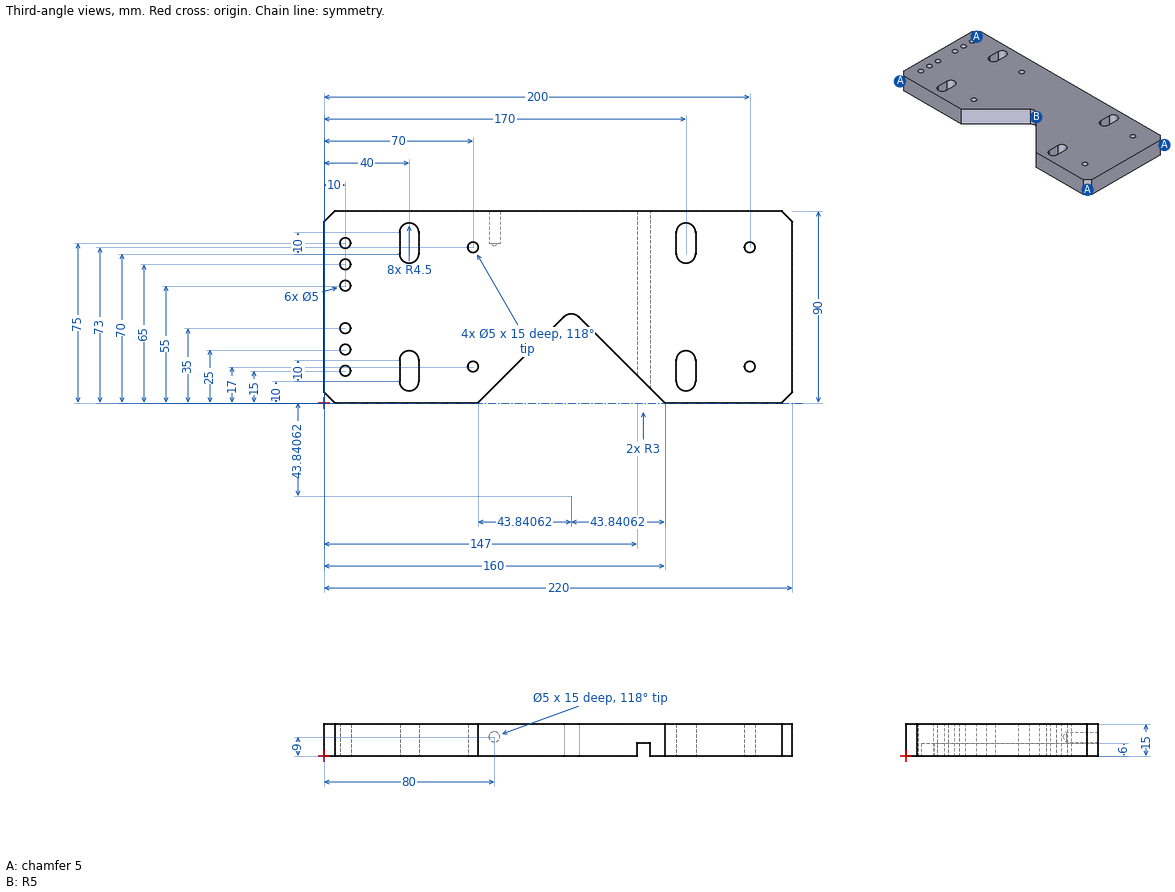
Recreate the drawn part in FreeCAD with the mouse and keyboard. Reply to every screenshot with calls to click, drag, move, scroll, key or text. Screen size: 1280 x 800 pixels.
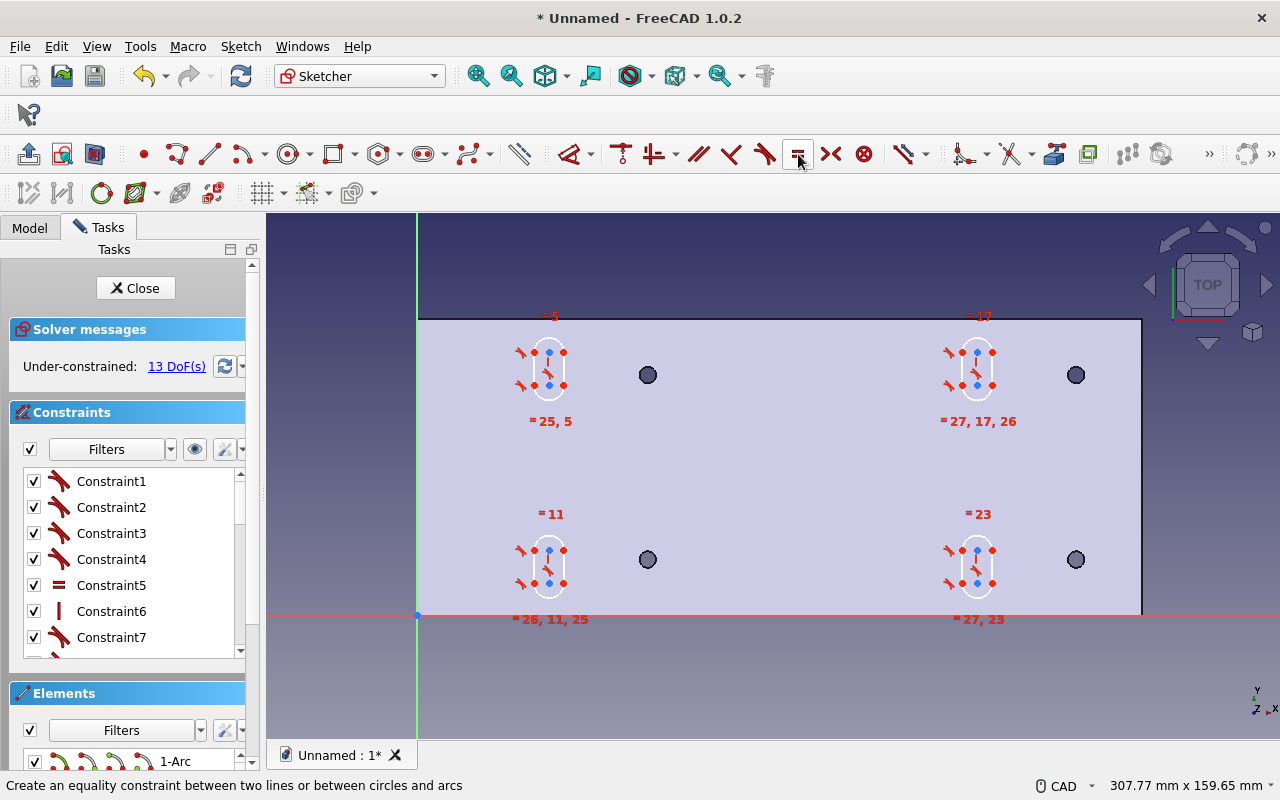
key(d)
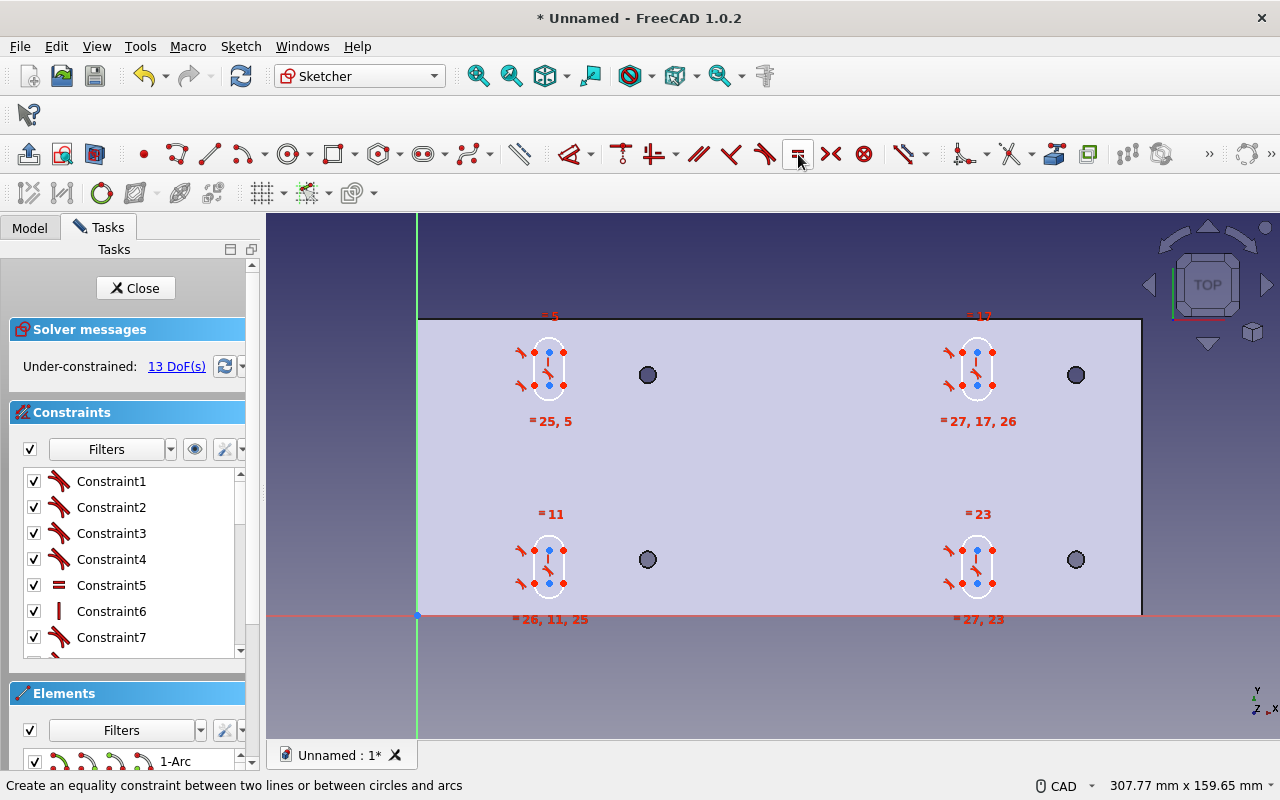
scroll(540, 398, up, 5)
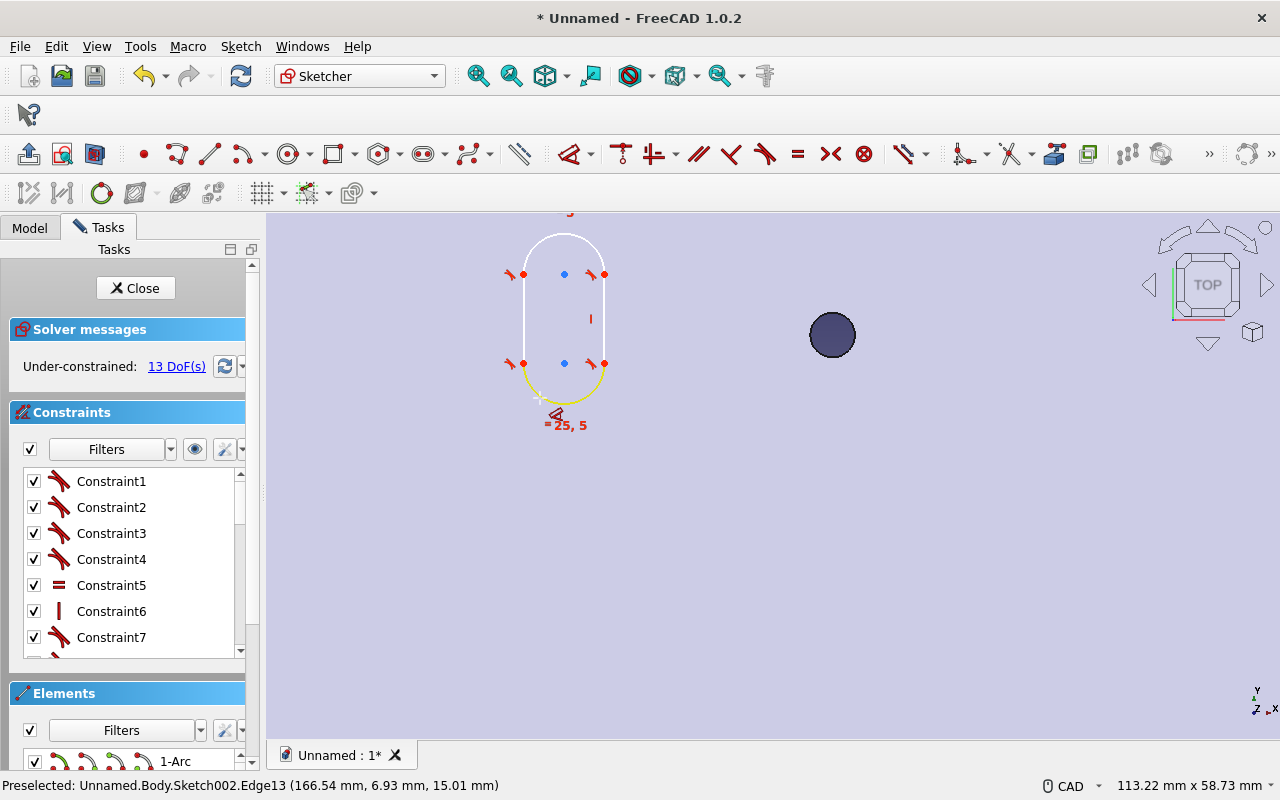
click(540, 396)
click(521, 422)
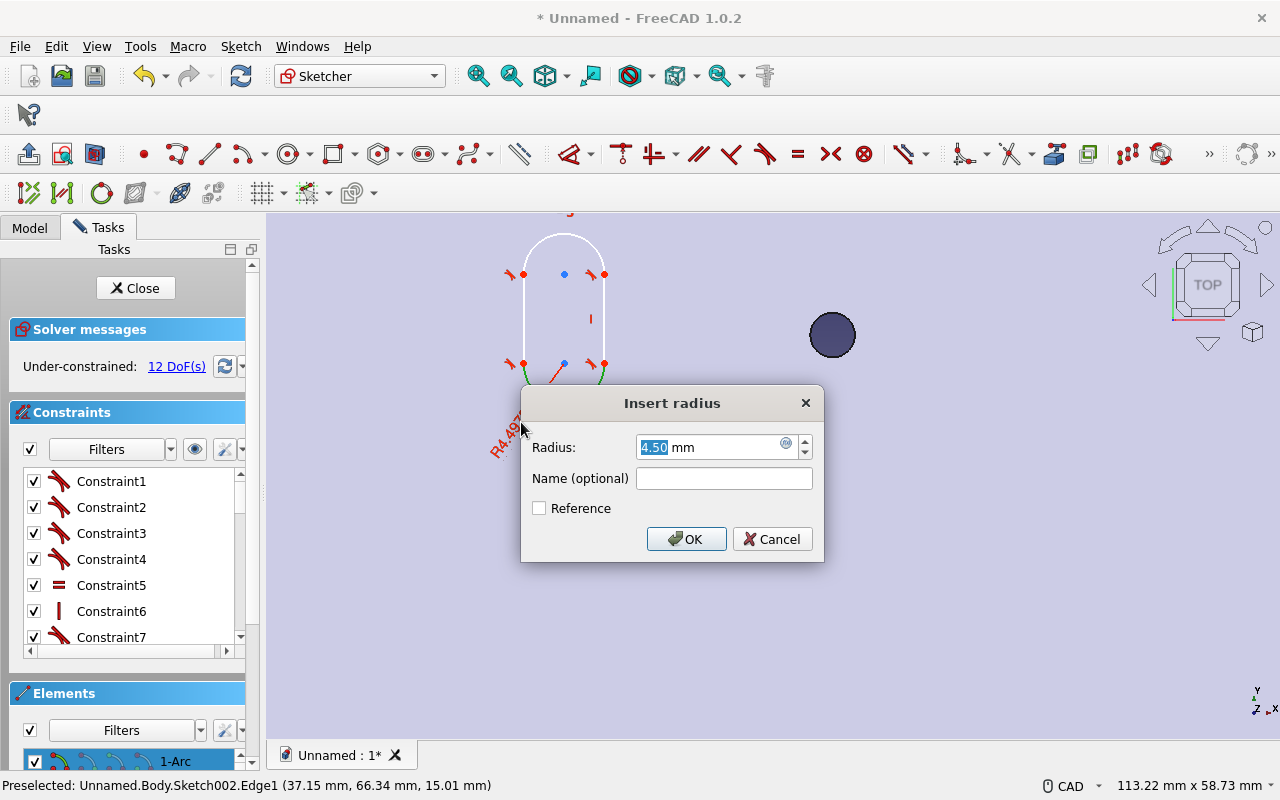
text(4.5)
key(Return)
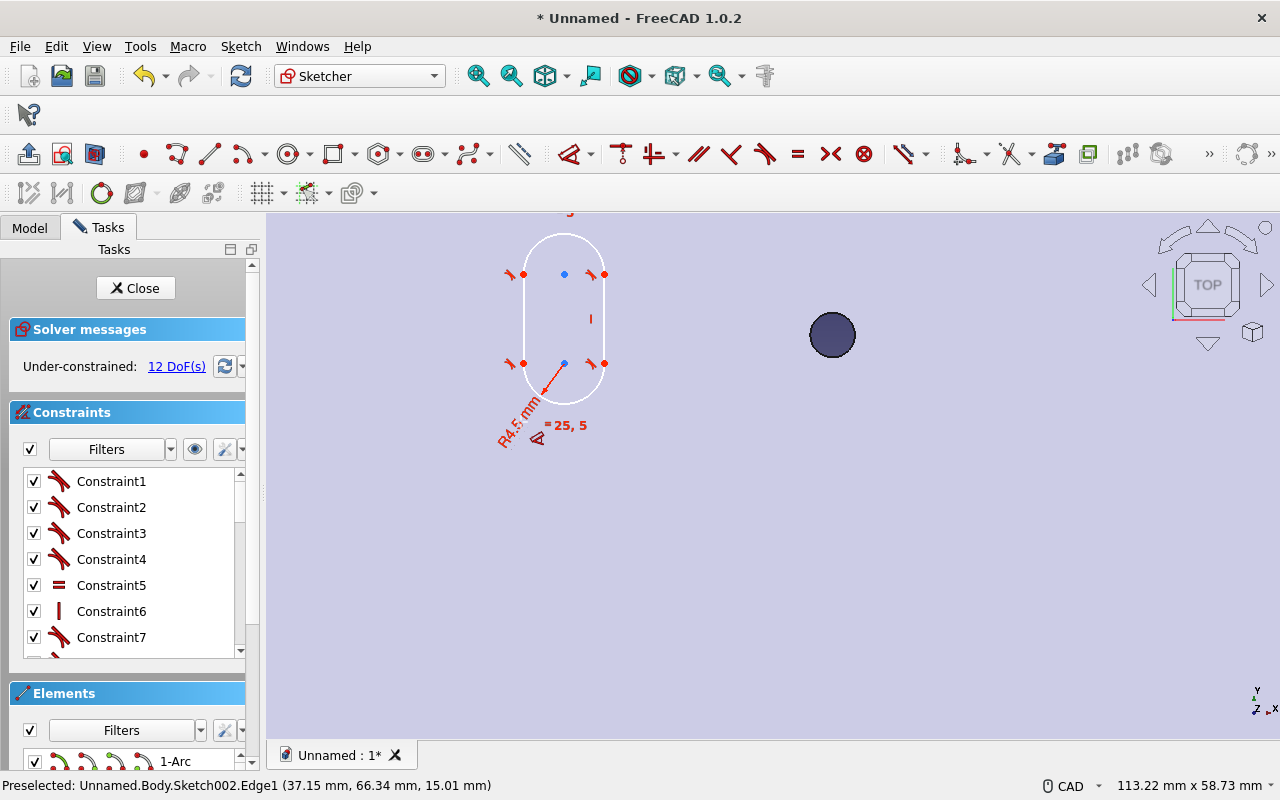
click(524, 337)
click(490, 319)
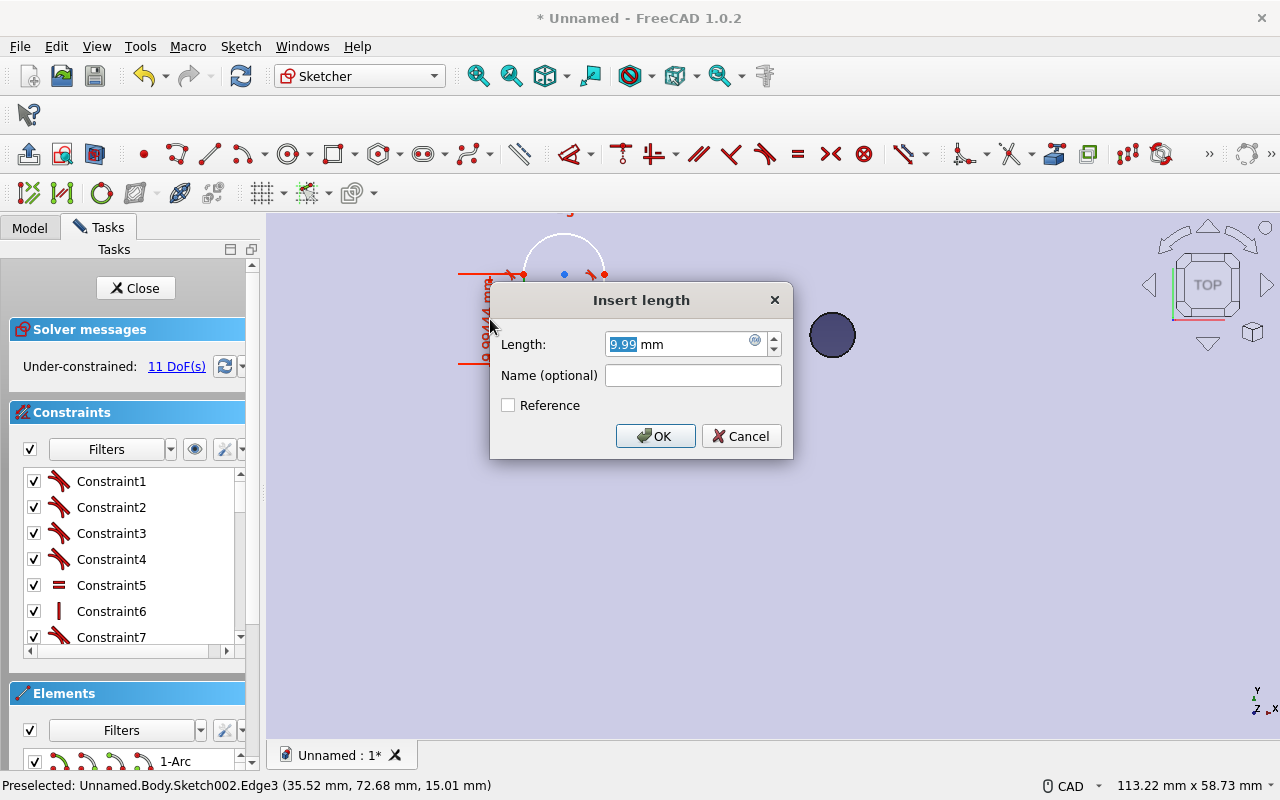
text(10)
key(Return)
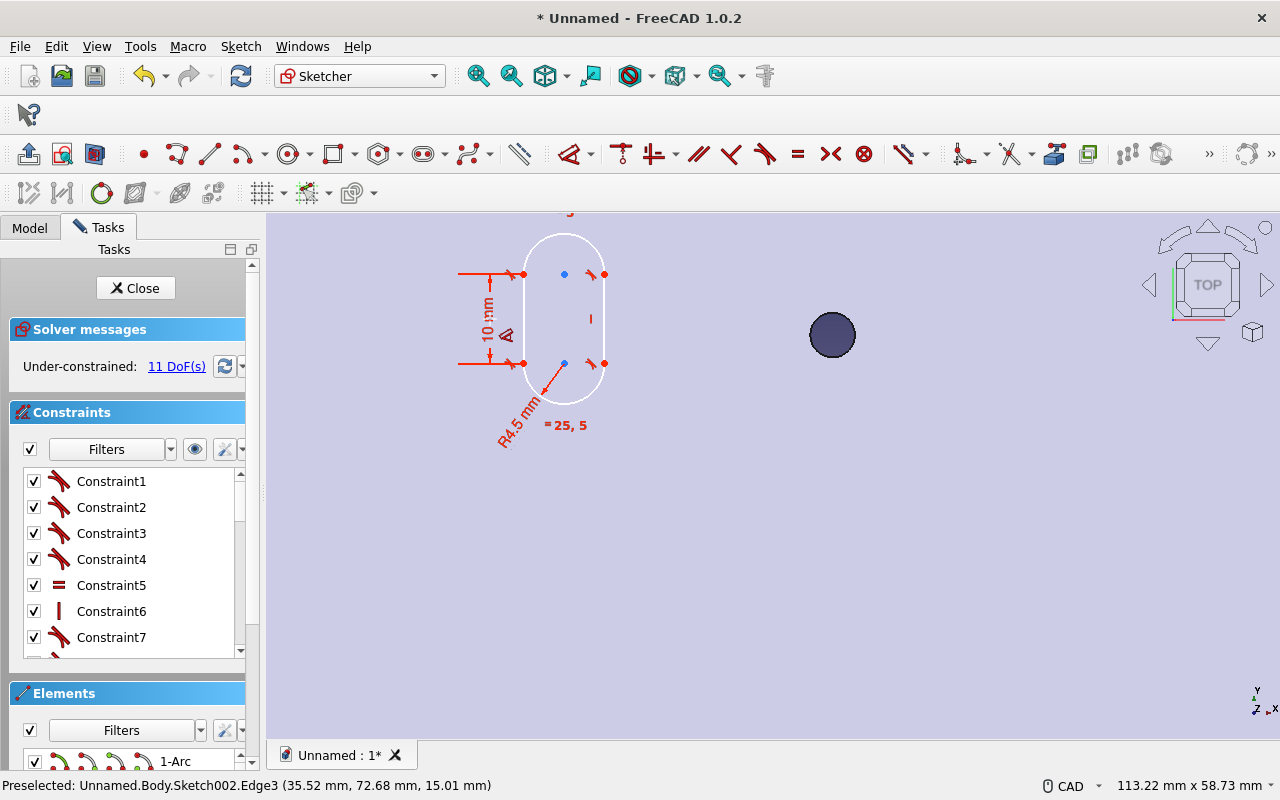
scroll(540, 398, down, 5)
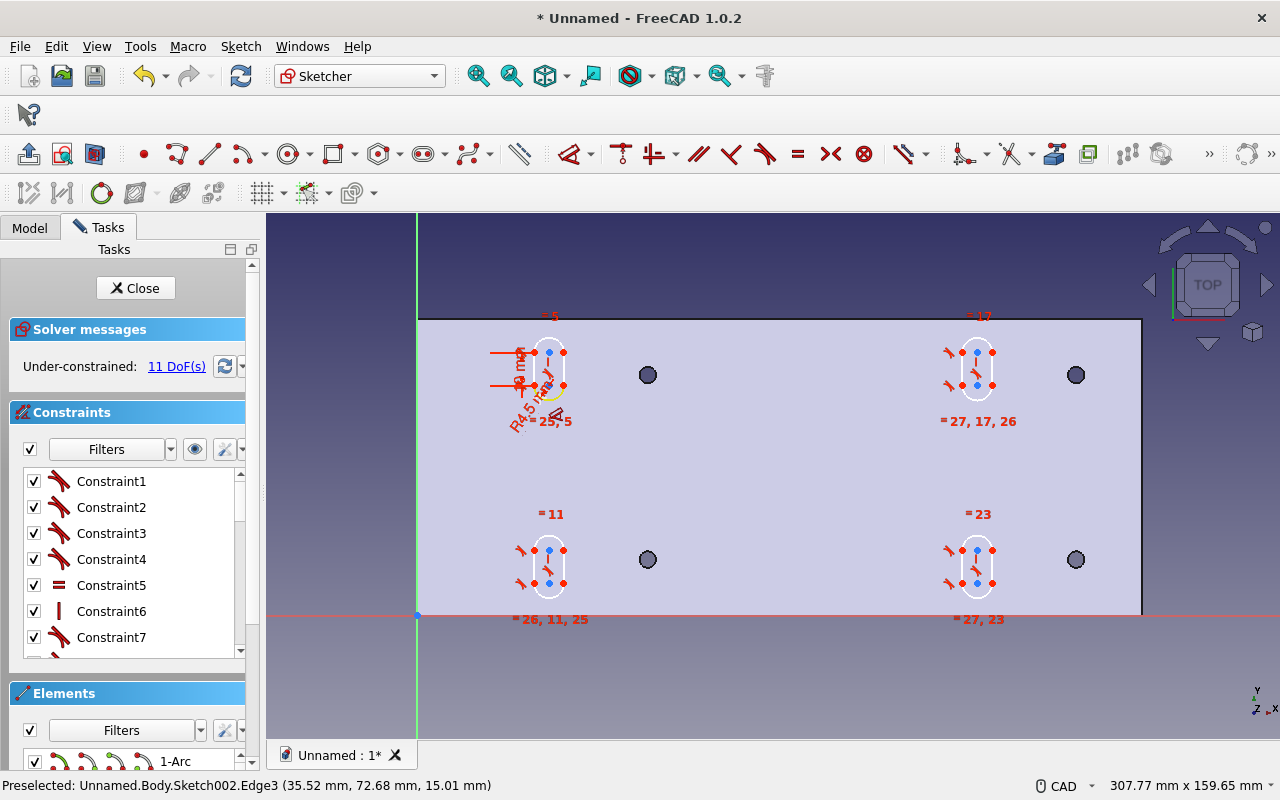
scroll(534, 573, up, 2)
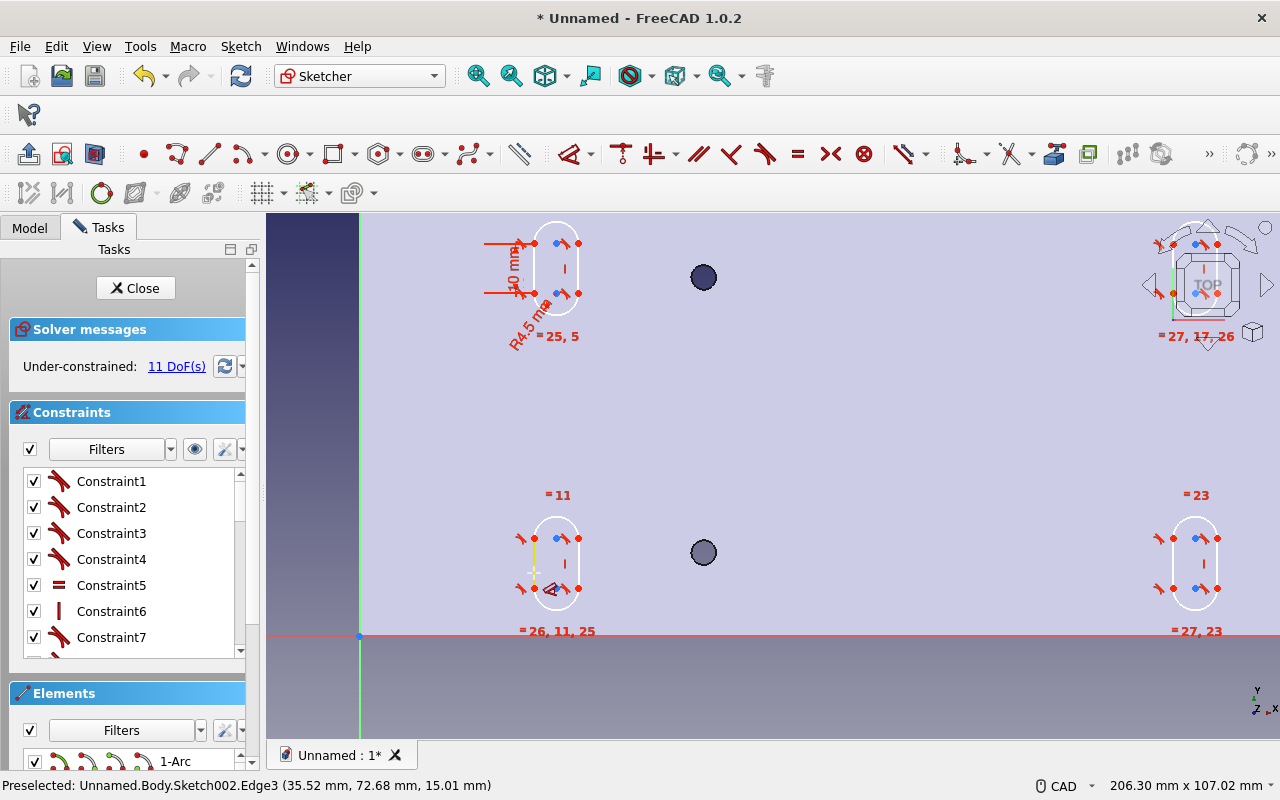
click(534, 573)
click(500, 563)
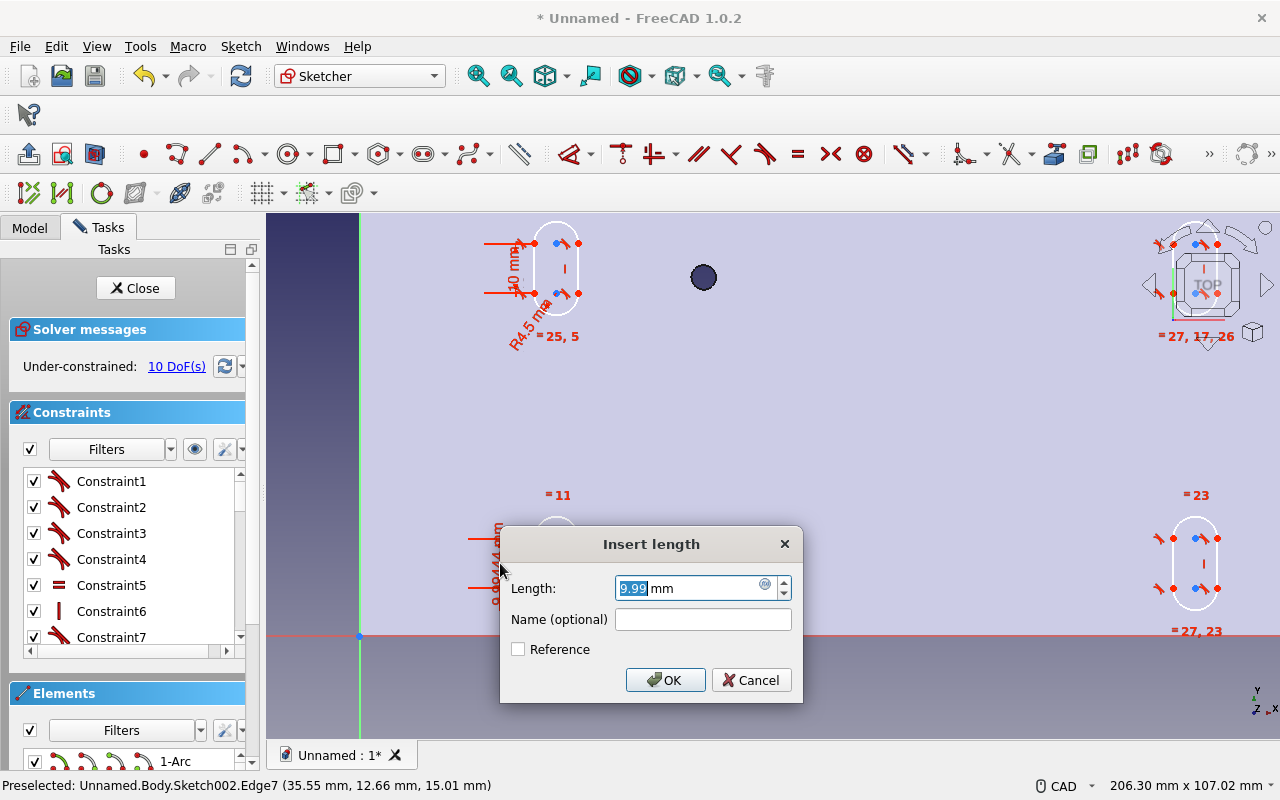
text(10)
key(Return)